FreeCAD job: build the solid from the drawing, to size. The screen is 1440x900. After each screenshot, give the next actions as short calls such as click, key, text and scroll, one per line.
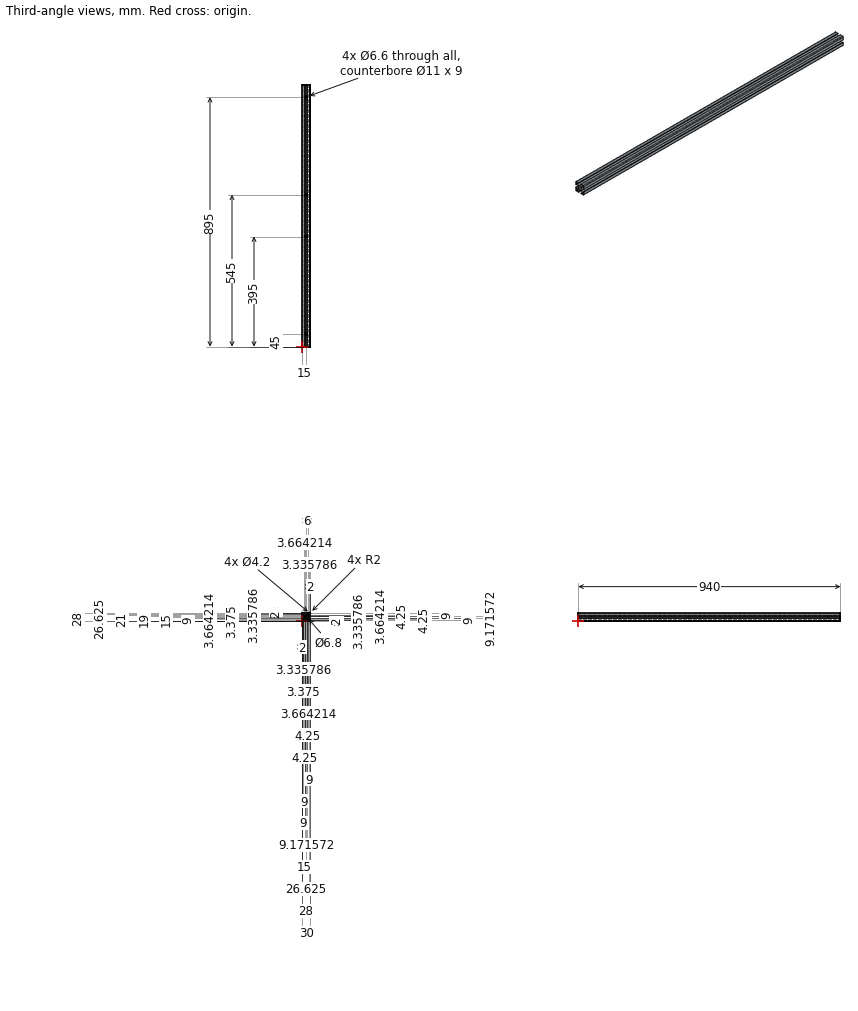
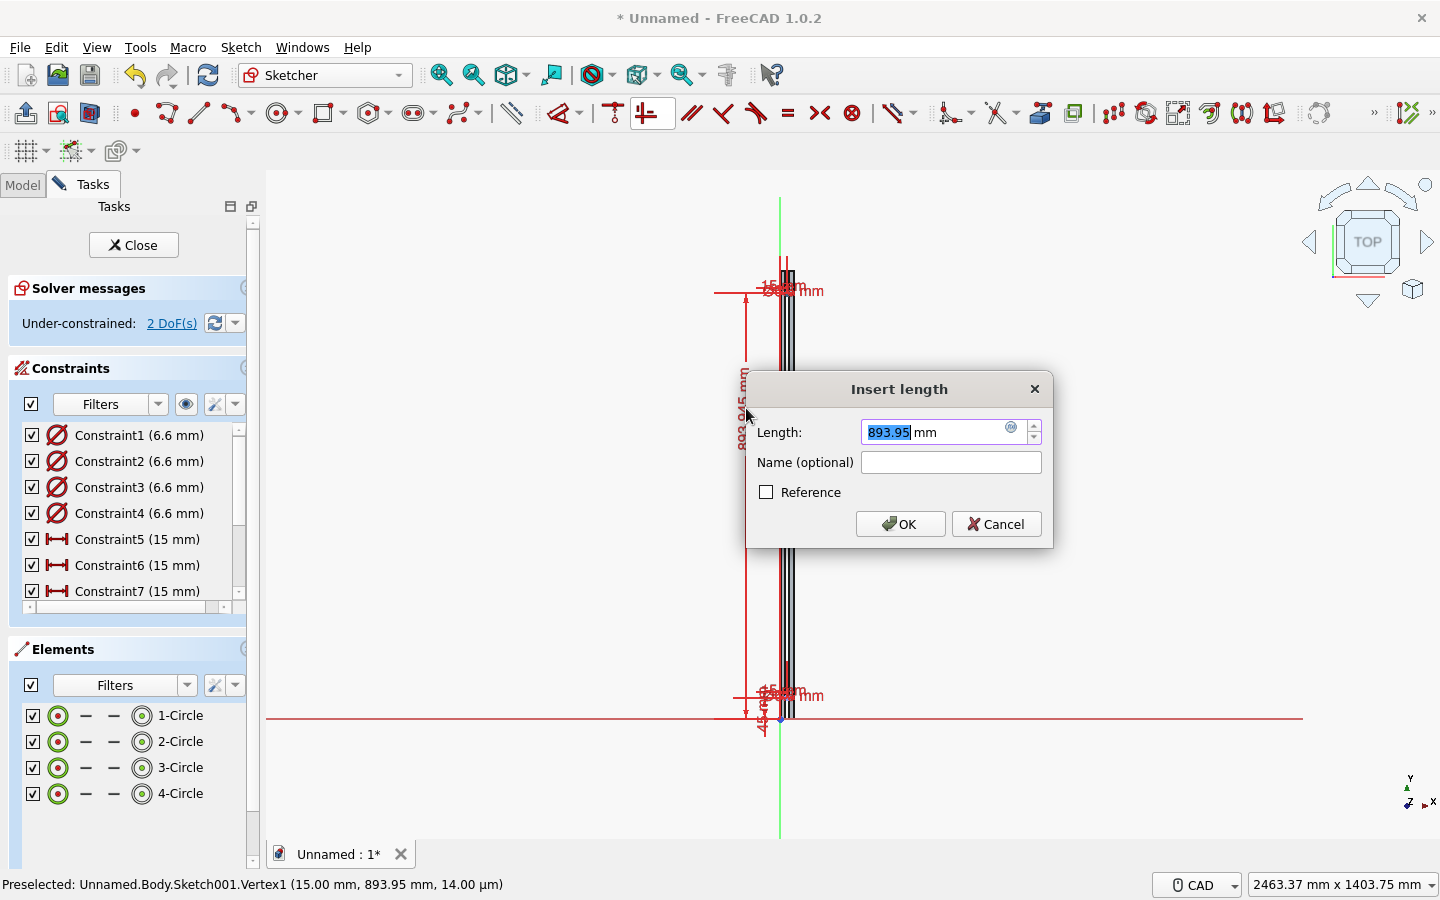
text(895)
key(Return)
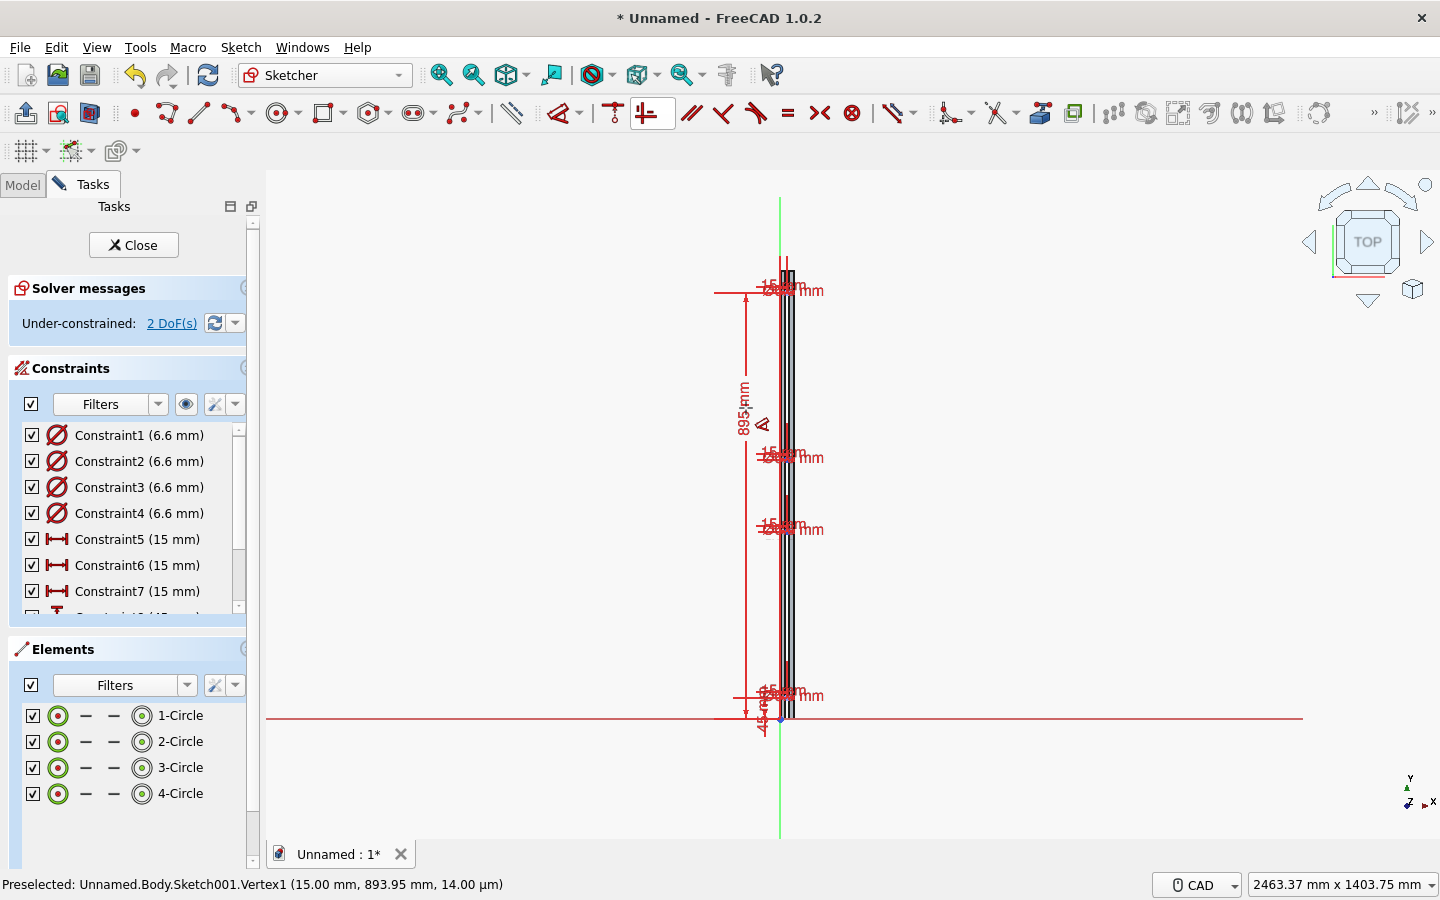
click(787, 460)
click(746, 590)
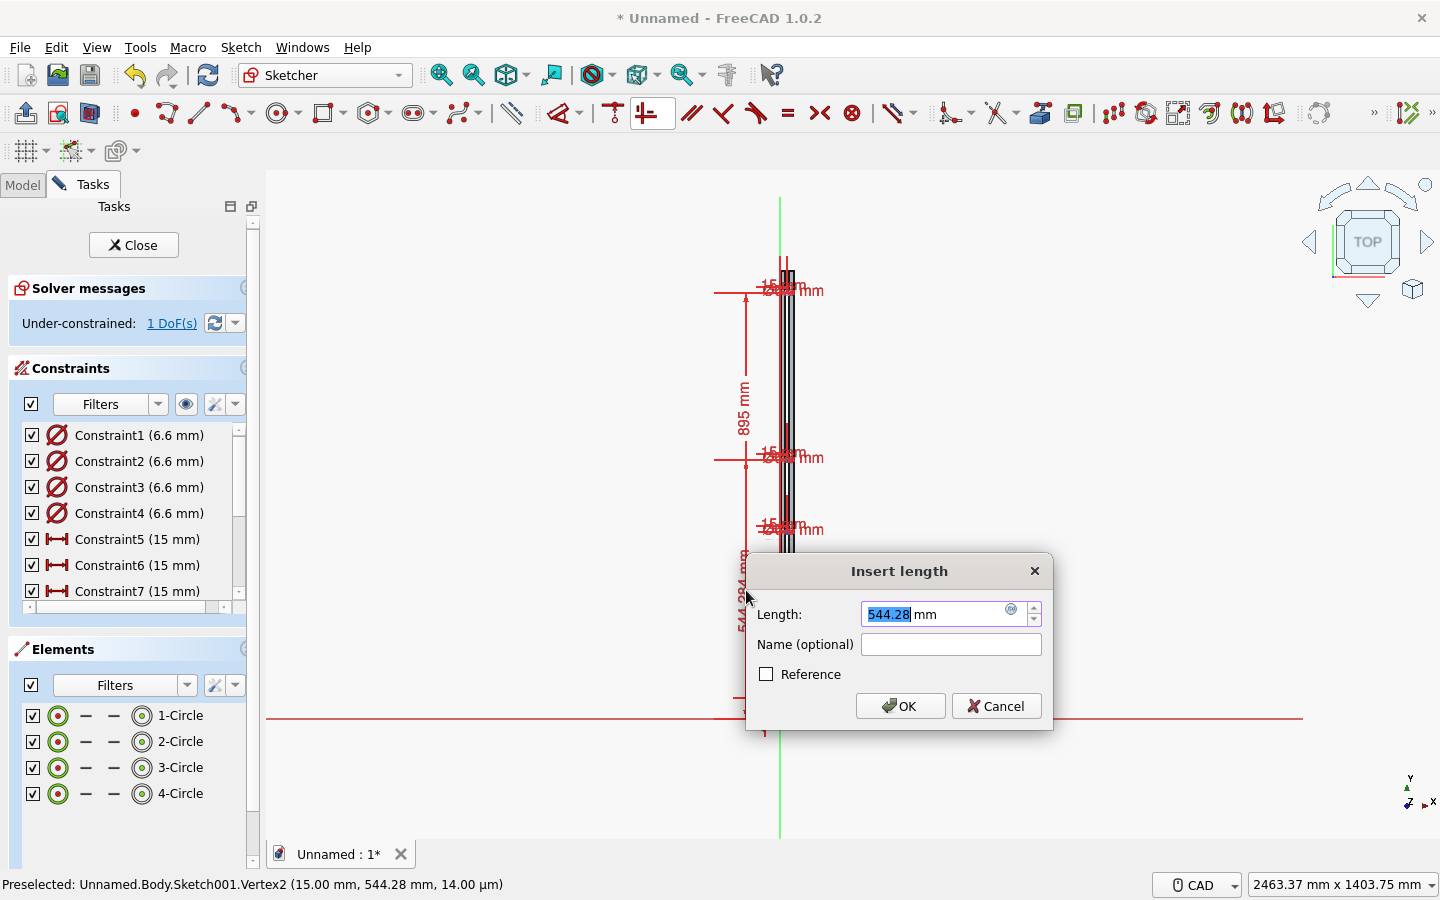
text(545)
key(Return)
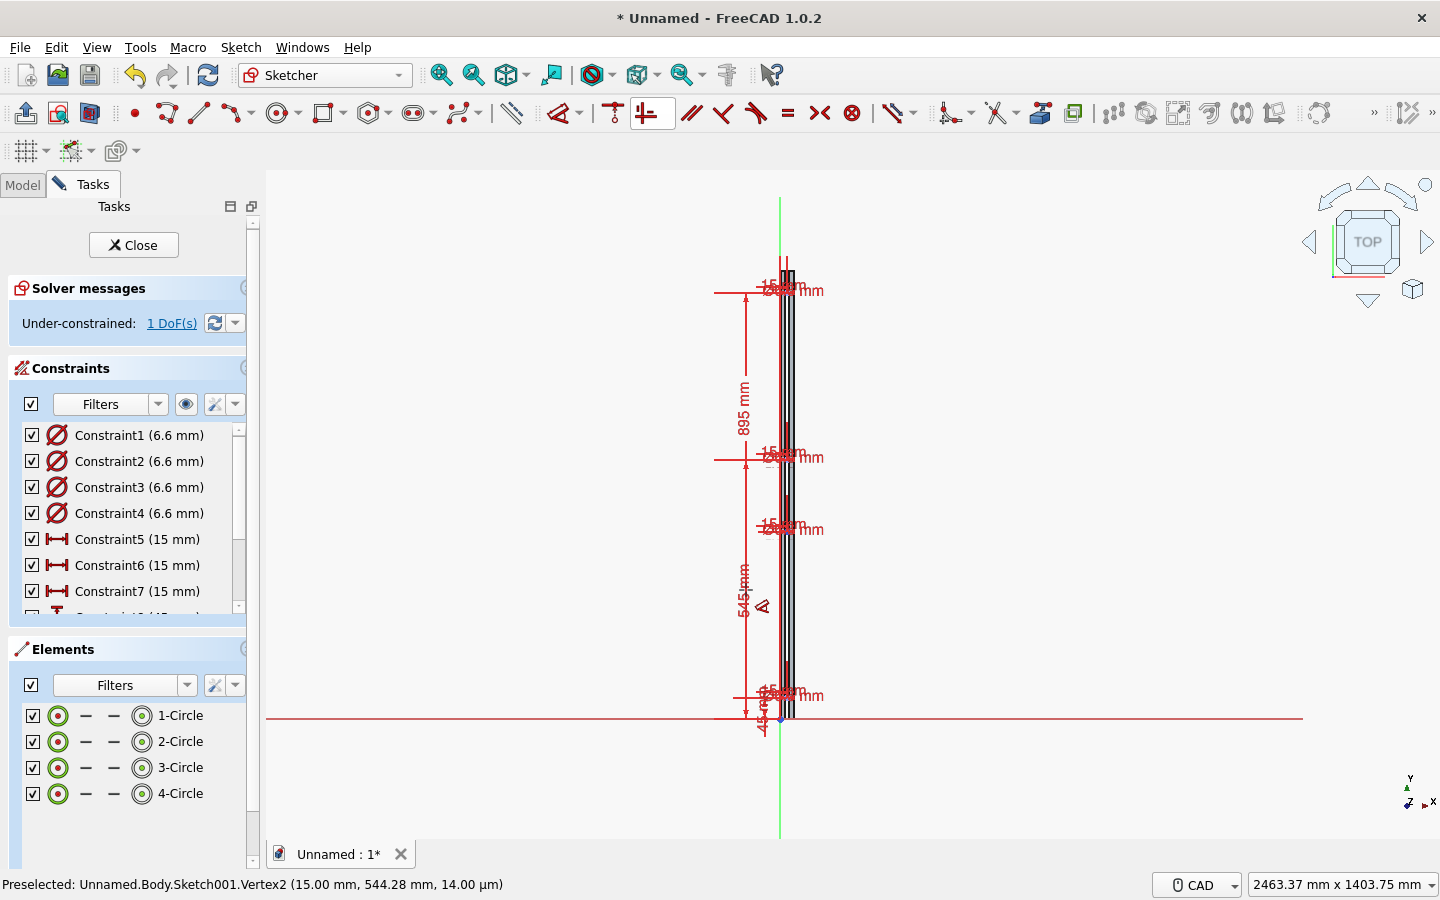
click(787, 532)
click(746, 625)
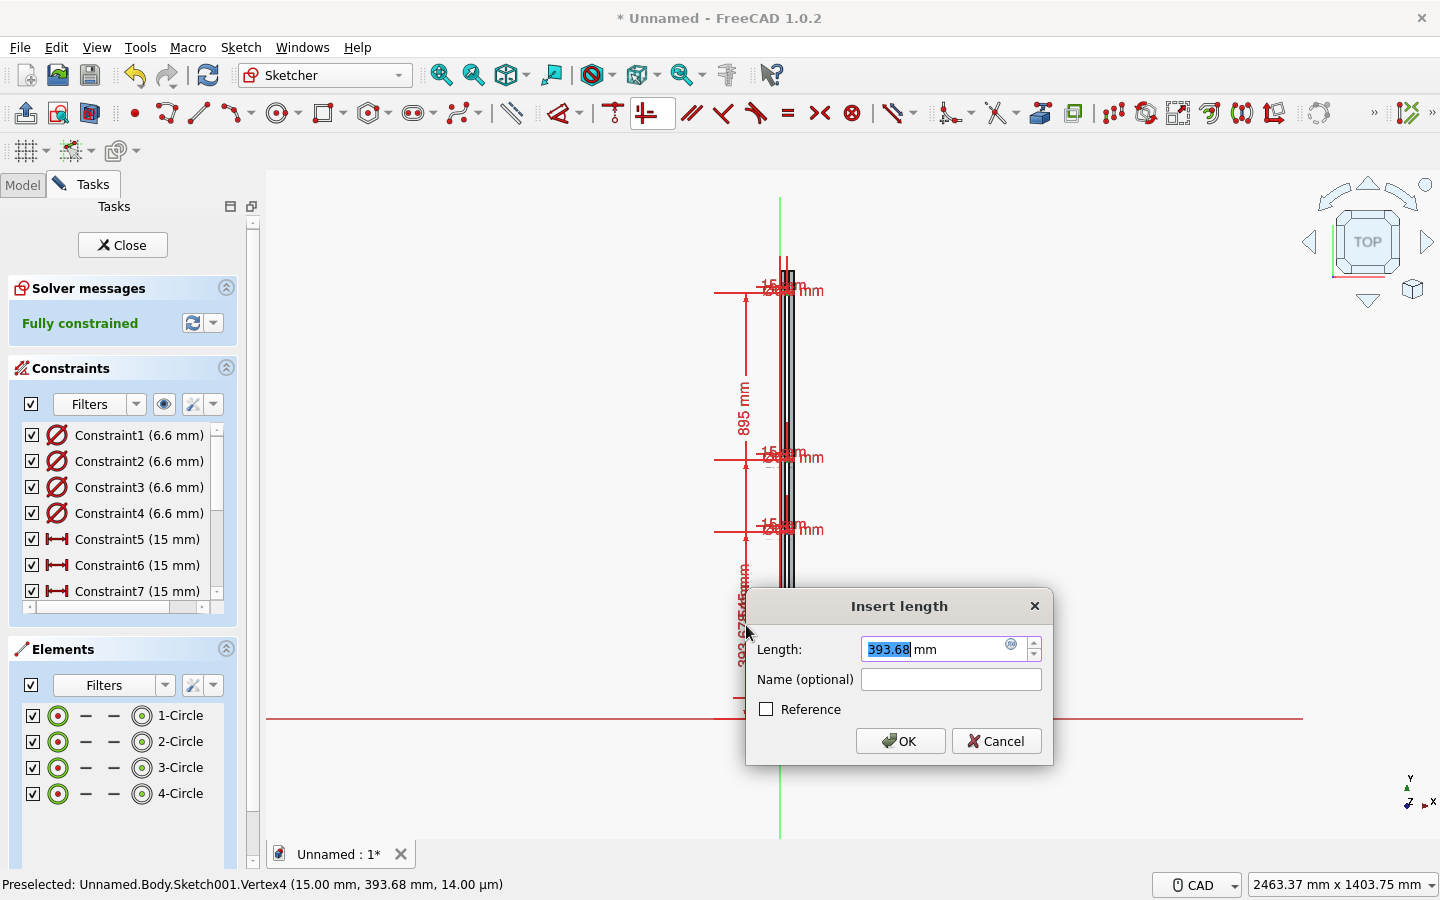
text(395)
key(Return)
key(Escape)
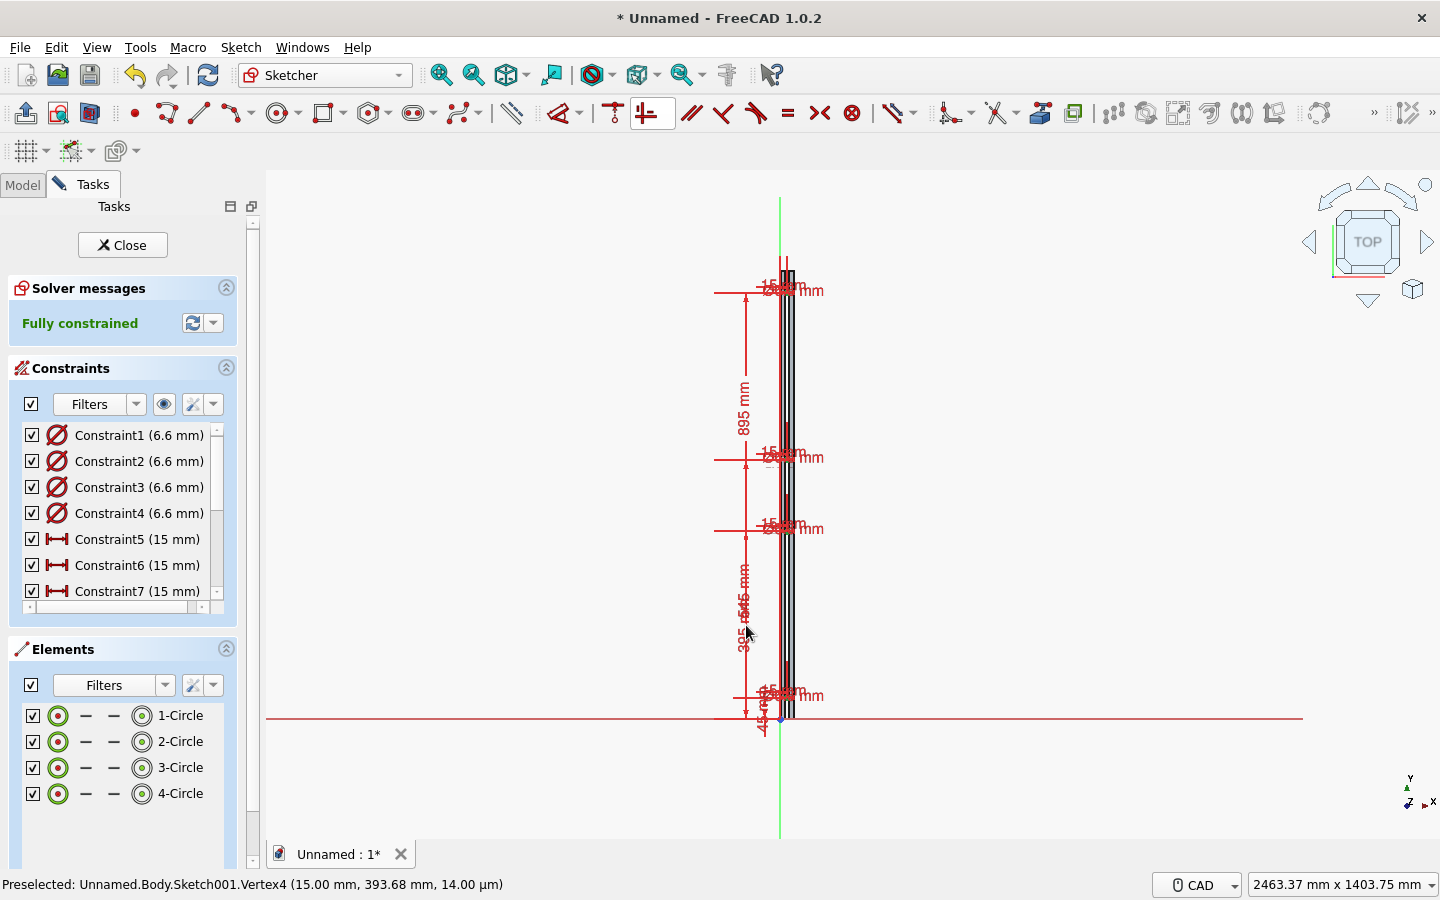
click(123, 245)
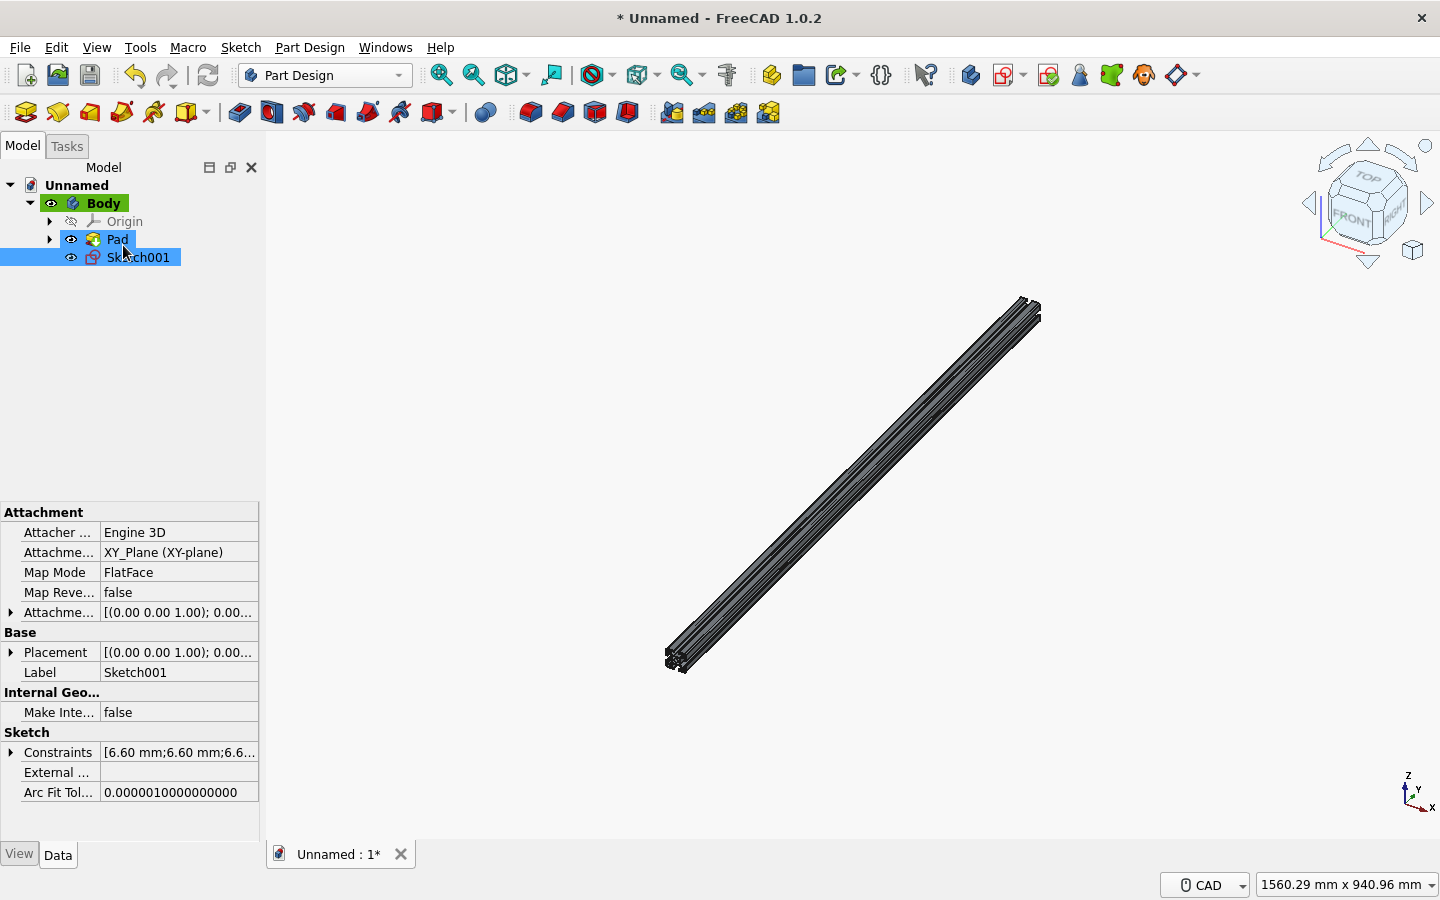
click(272, 112)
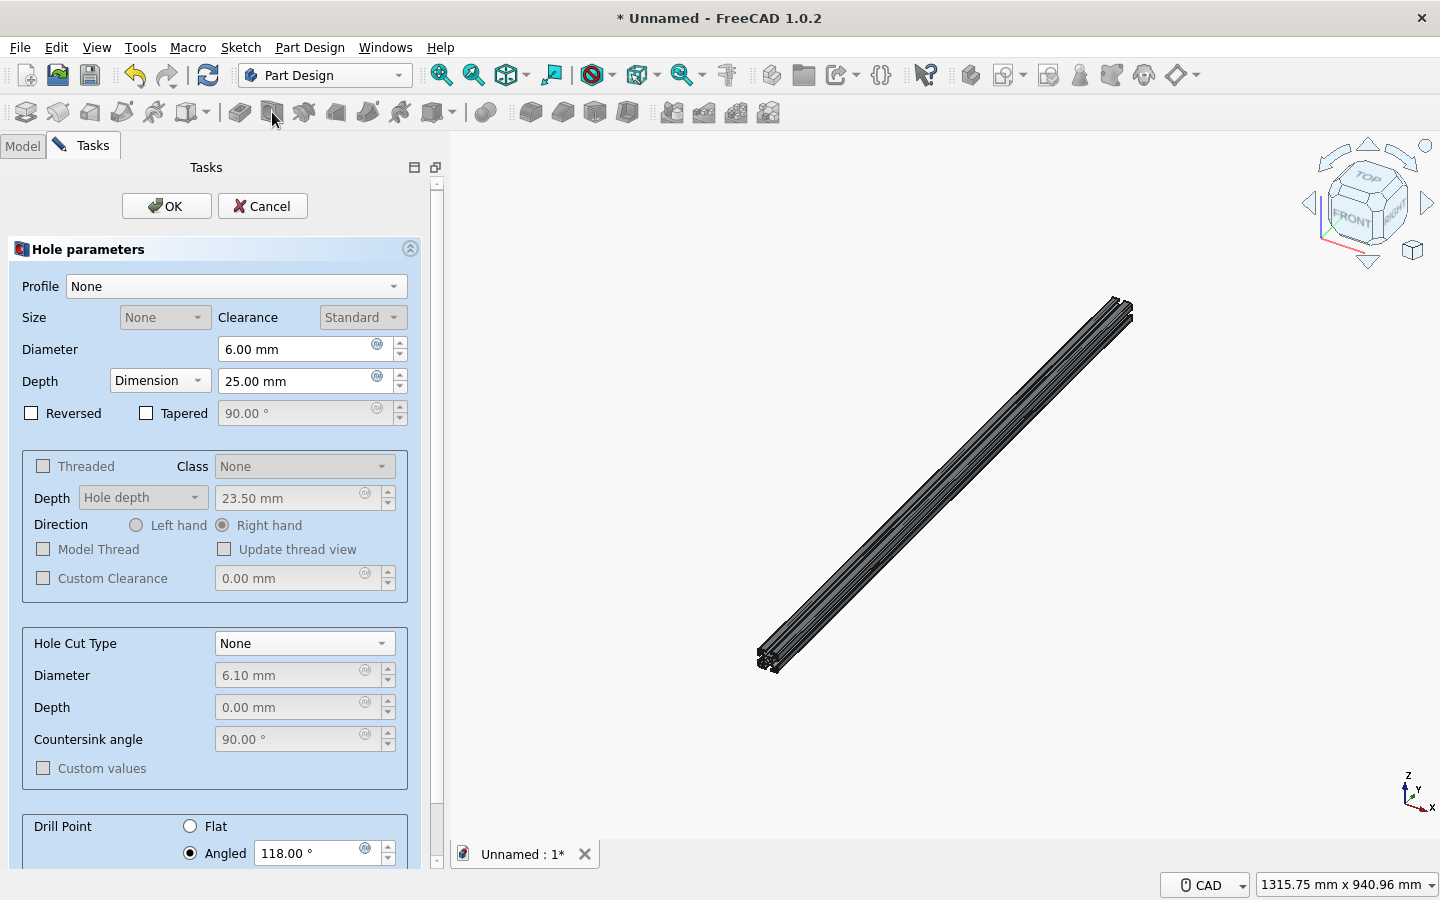
triple_click(305, 349)